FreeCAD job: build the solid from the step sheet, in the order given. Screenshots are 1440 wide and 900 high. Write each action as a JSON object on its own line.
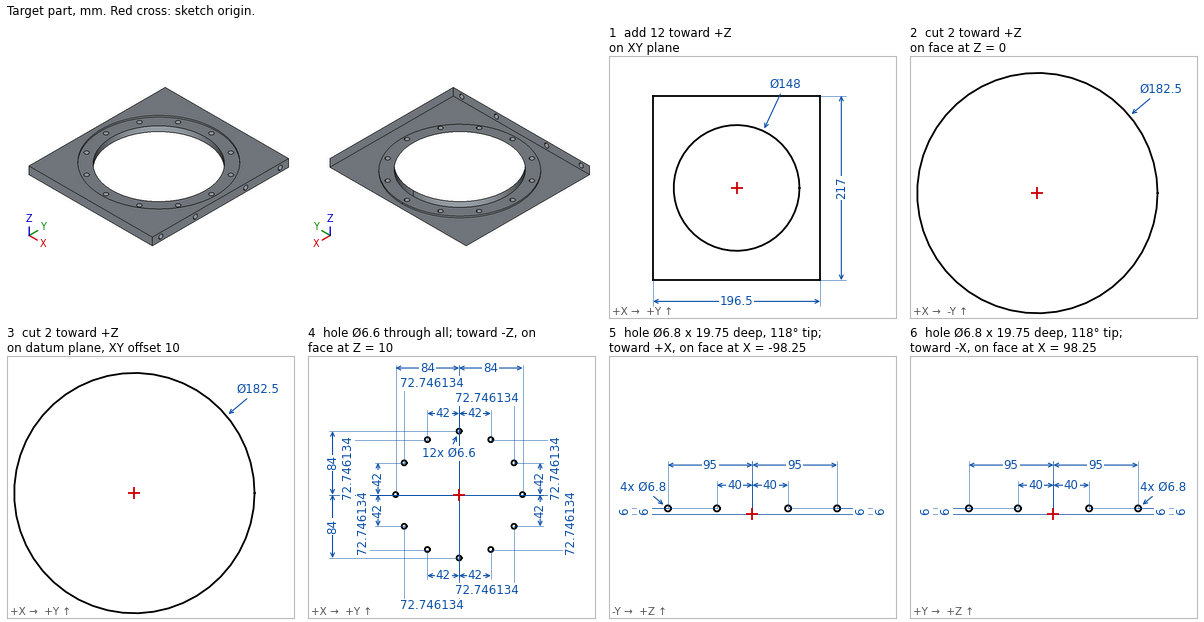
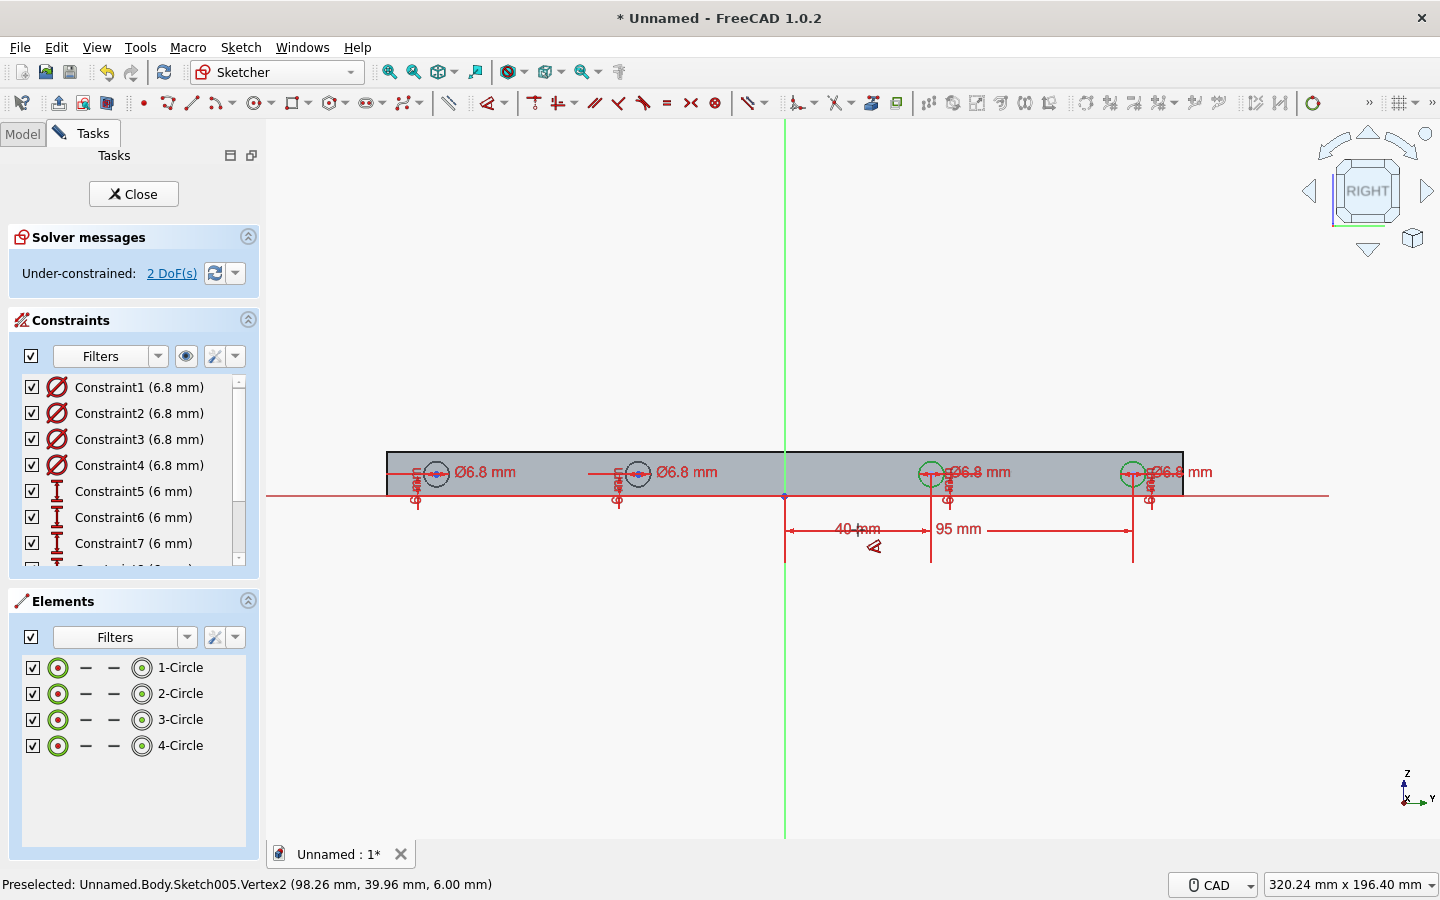
{"action": "left_click", "coordinate": [638, 474]}
{"action": "left_click", "coordinate": [711, 530]}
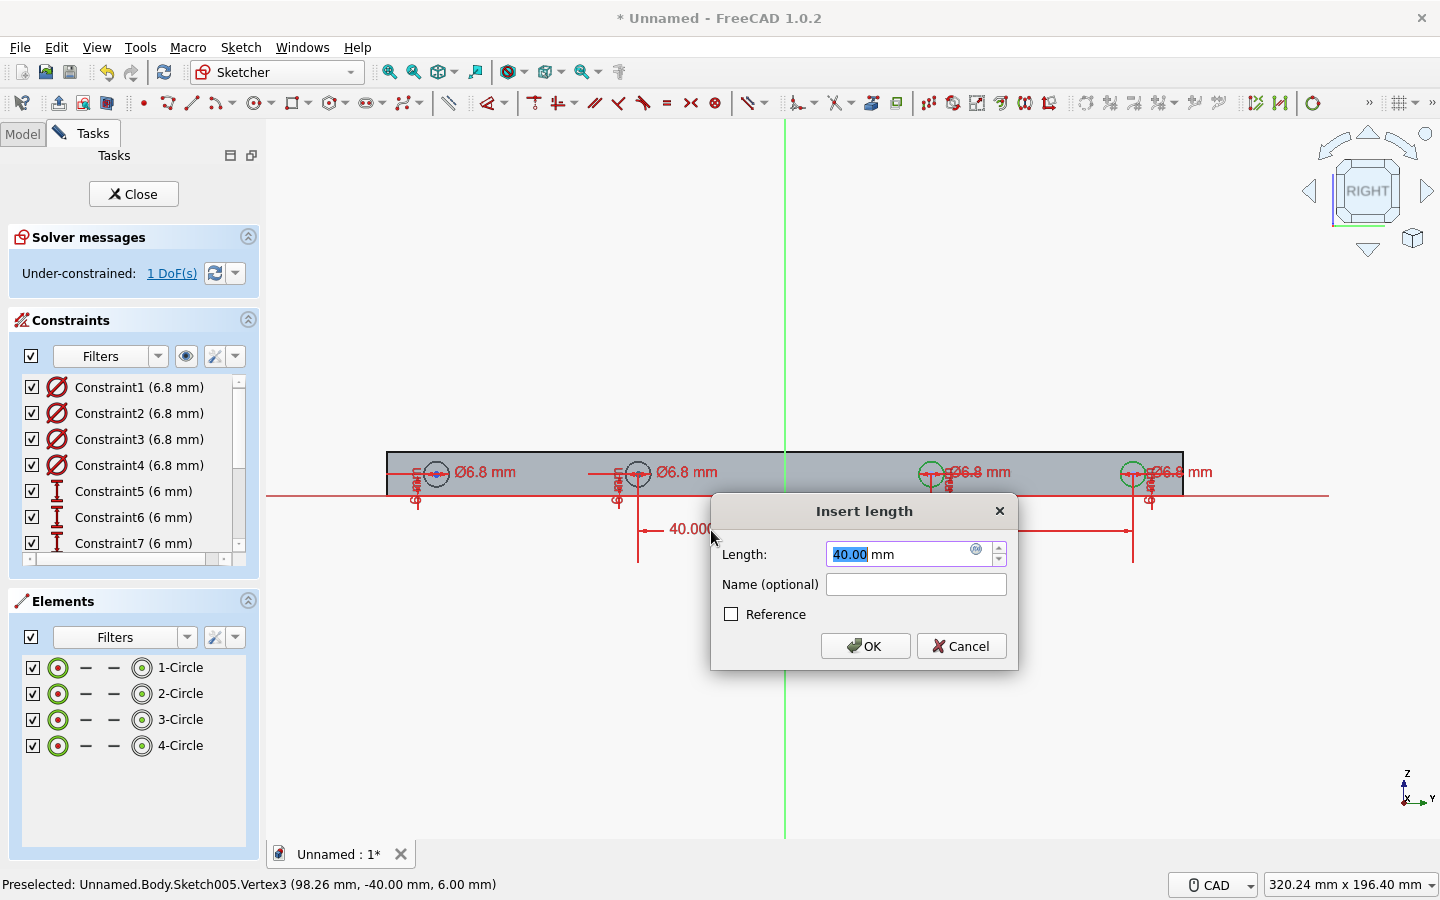
{"action": "type", "text": "40"}
{"action": "key", "text": "Return"}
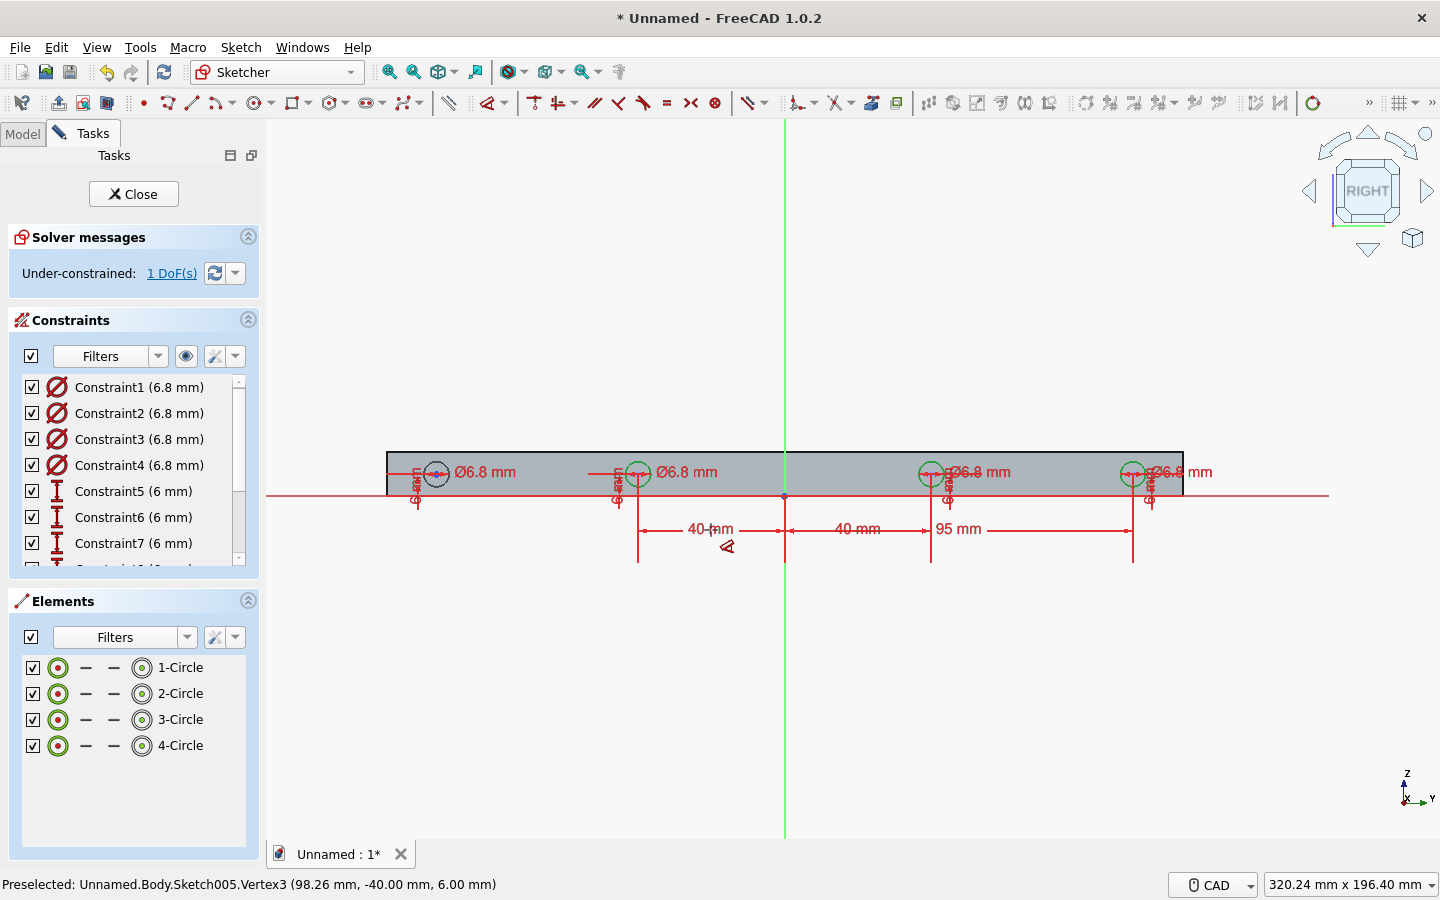
{"action": "left_click", "coordinate": [437, 474]}
{"action": "left_click", "coordinate": [611, 530]}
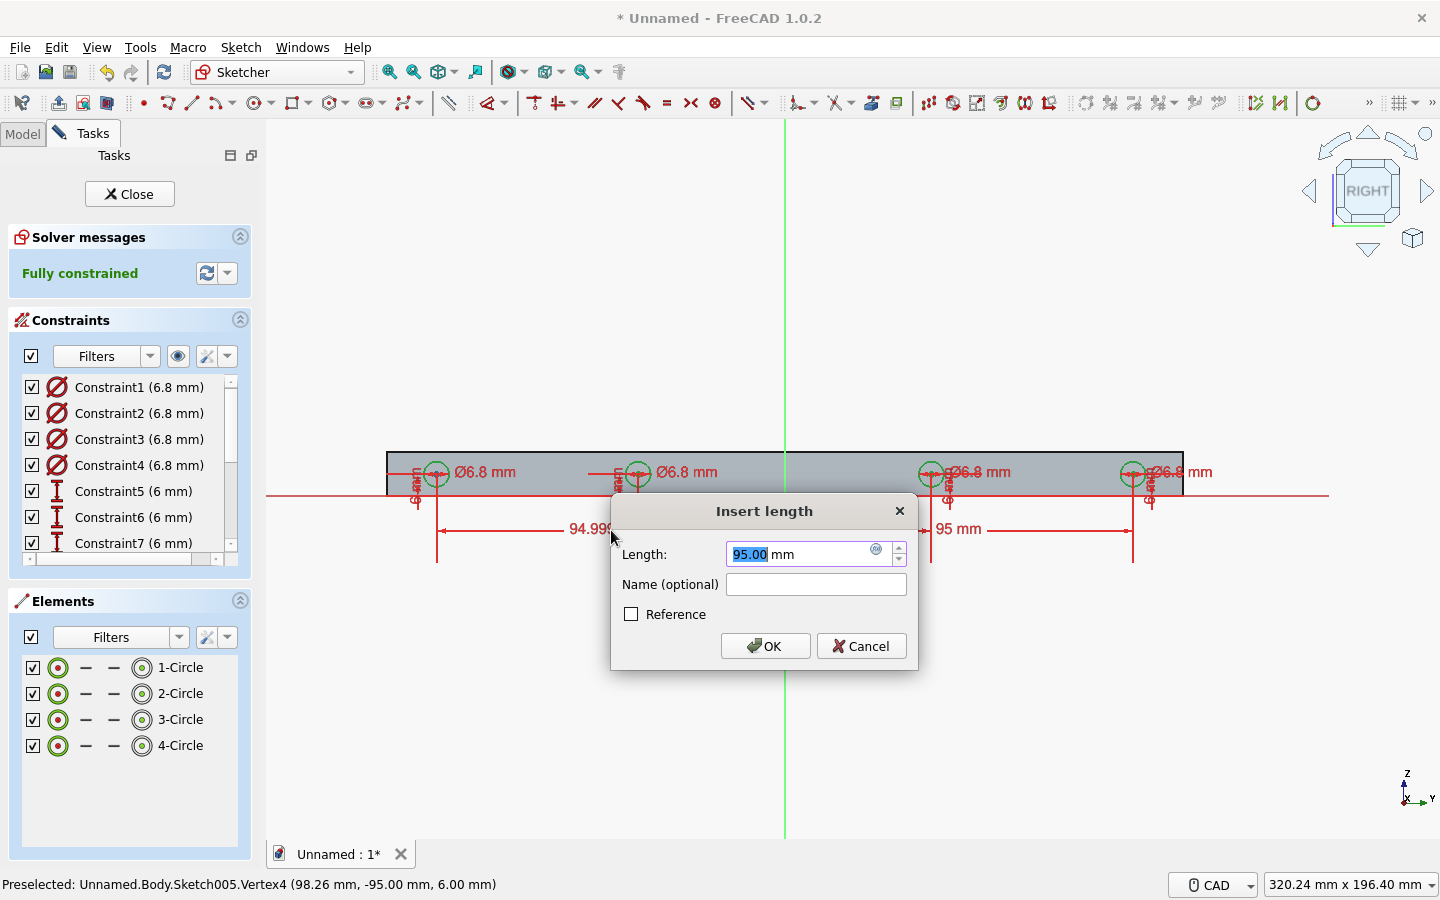
{"action": "type", "text": "95"}
{"action": "key", "text": "Return"}
{"action": "key", "text": "Escape"}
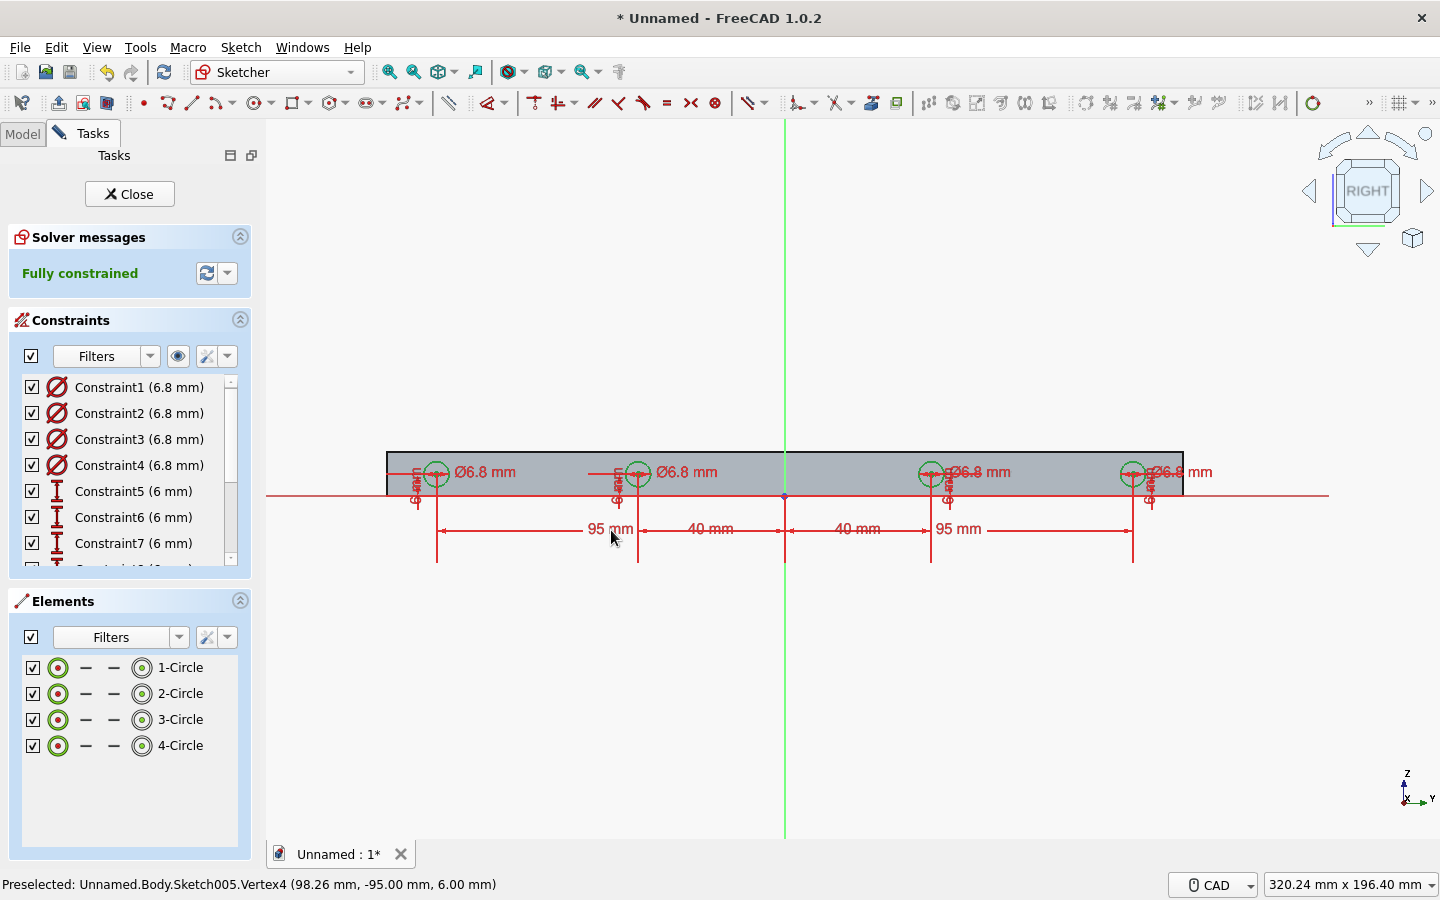
{"action": "left_click", "coordinate": [130, 194]}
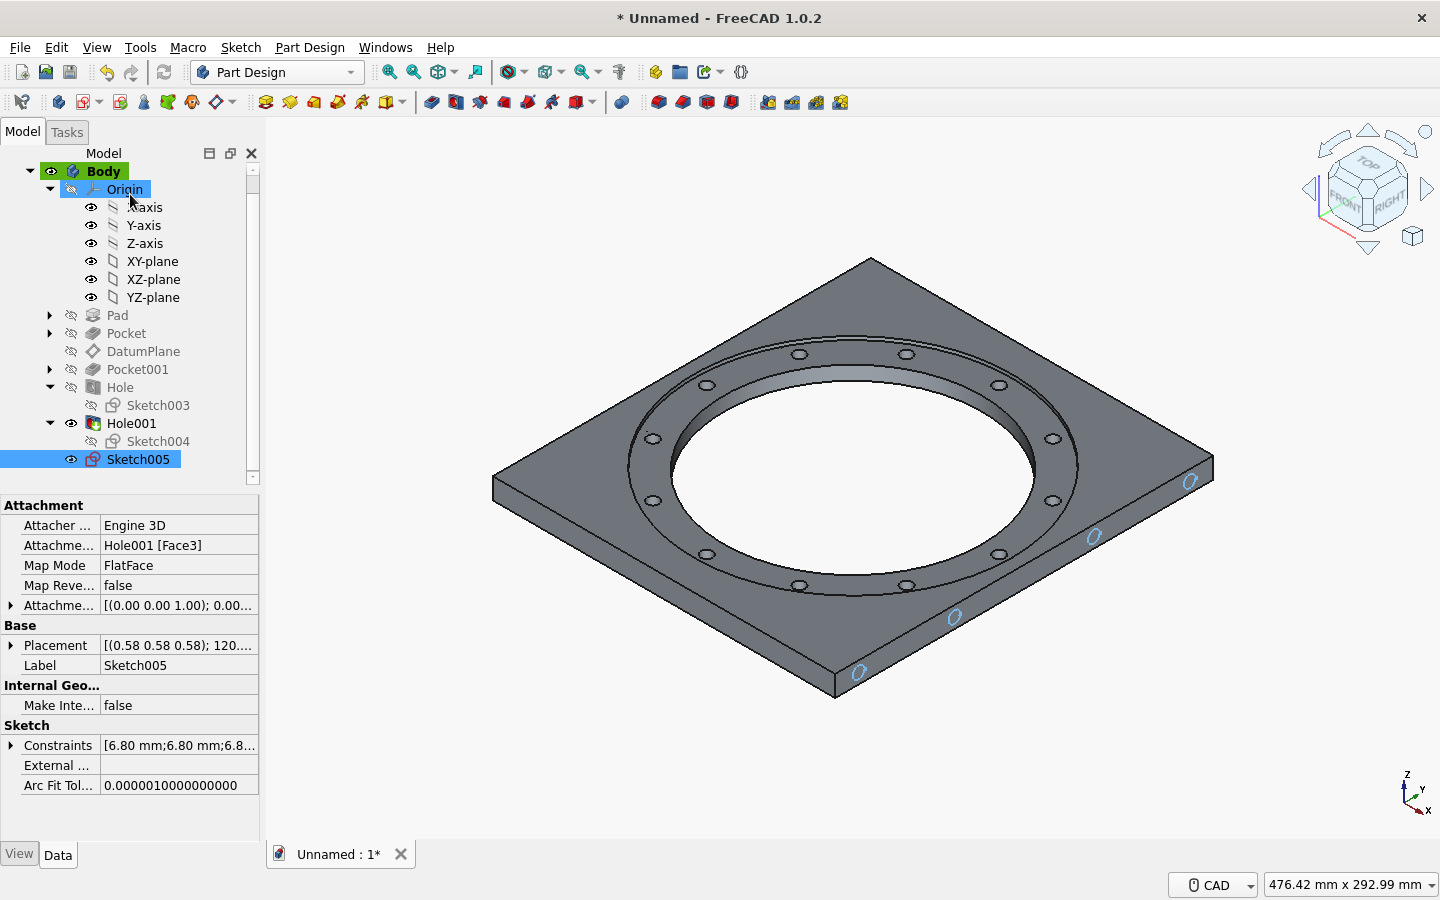
{"action": "left_click", "coordinate": [456, 102]}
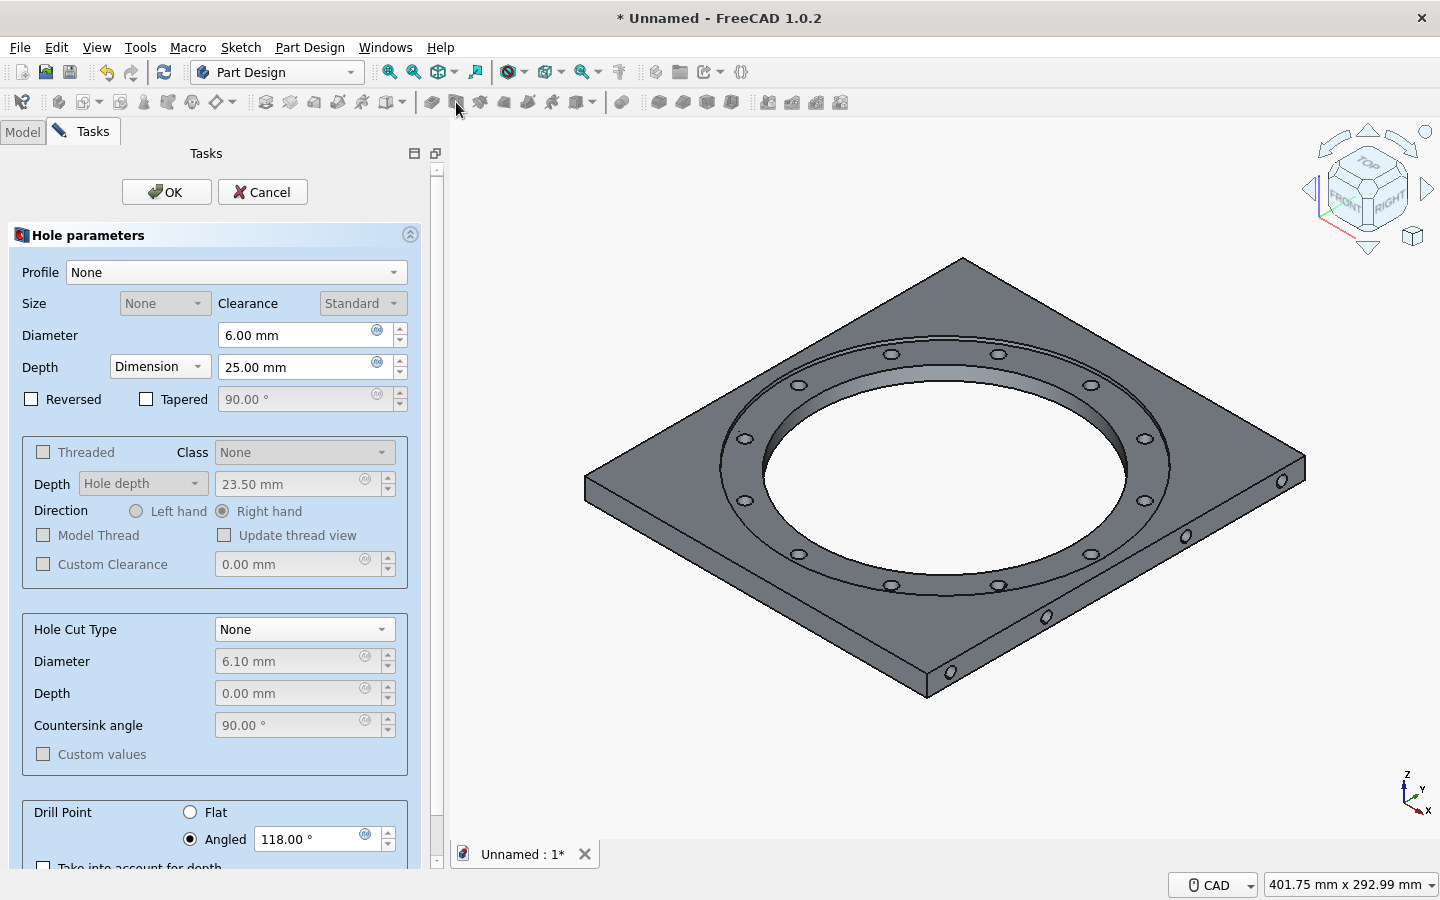
{"action": "triple_click", "coordinate": [305, 335]}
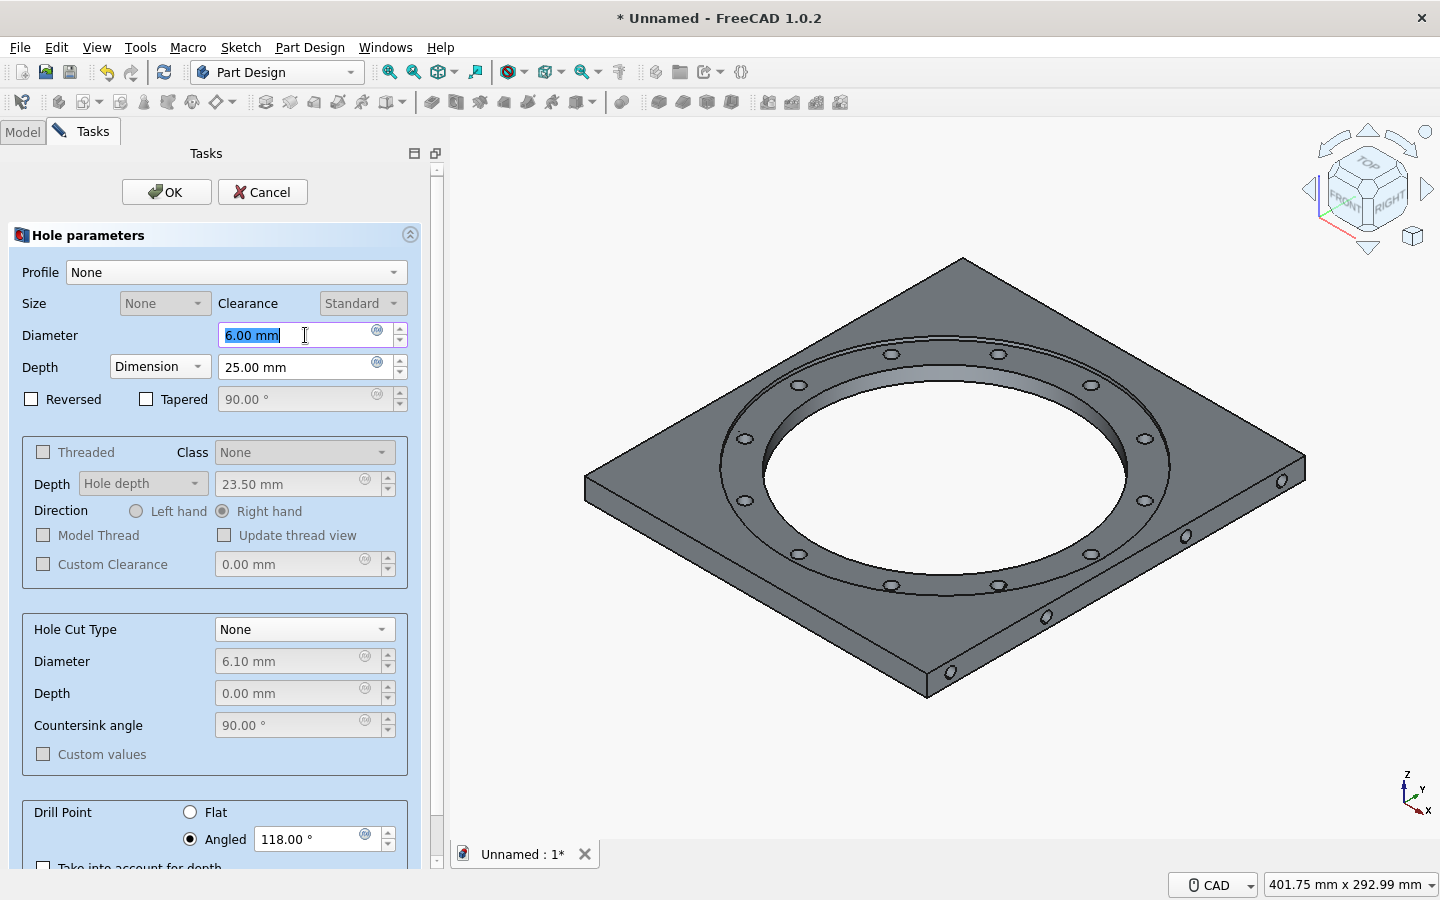
{"action": "type", "text": "6.8"}
{"action": "key", "text": "Tab"}